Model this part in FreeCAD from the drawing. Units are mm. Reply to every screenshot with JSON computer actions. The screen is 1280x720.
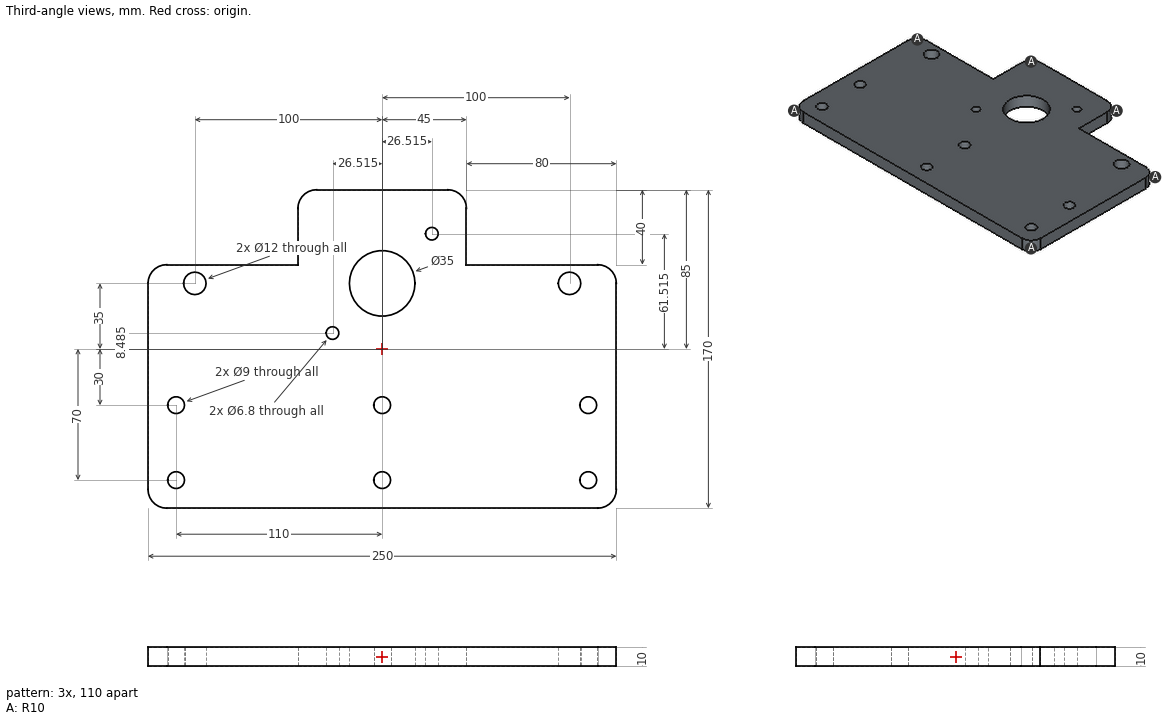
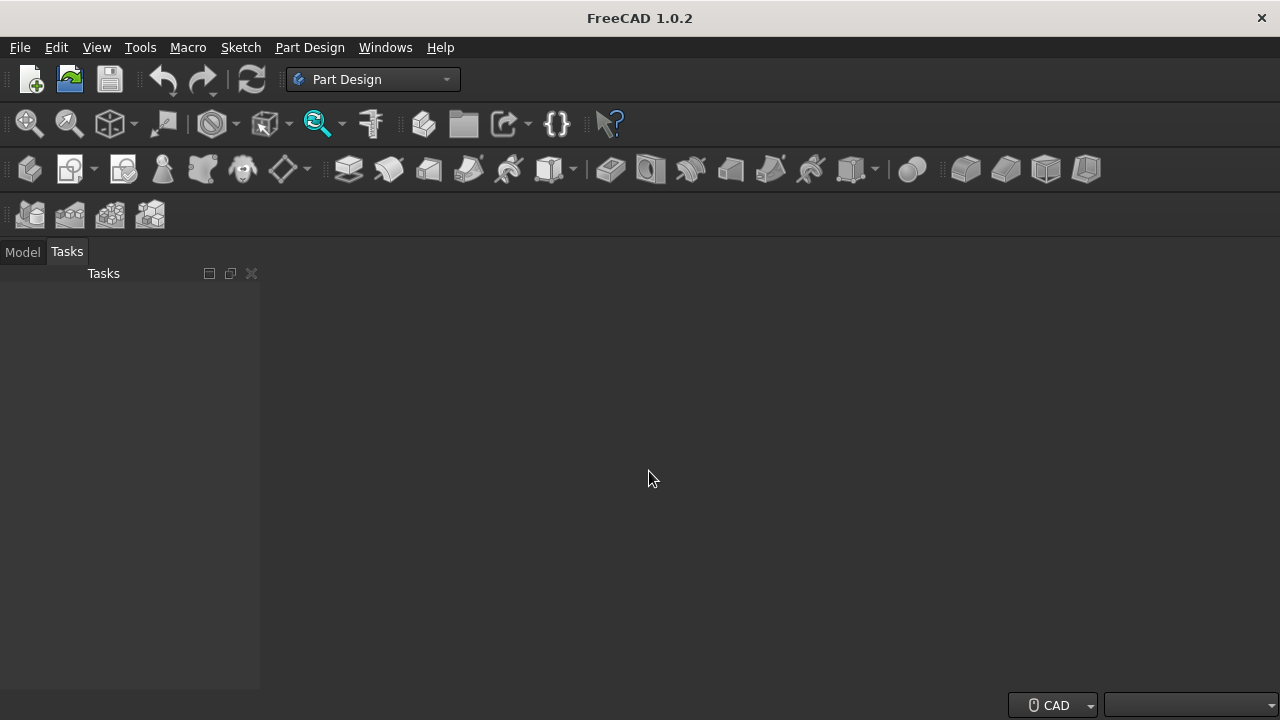
{"action": "left_click", "coordinate": [30, 80]}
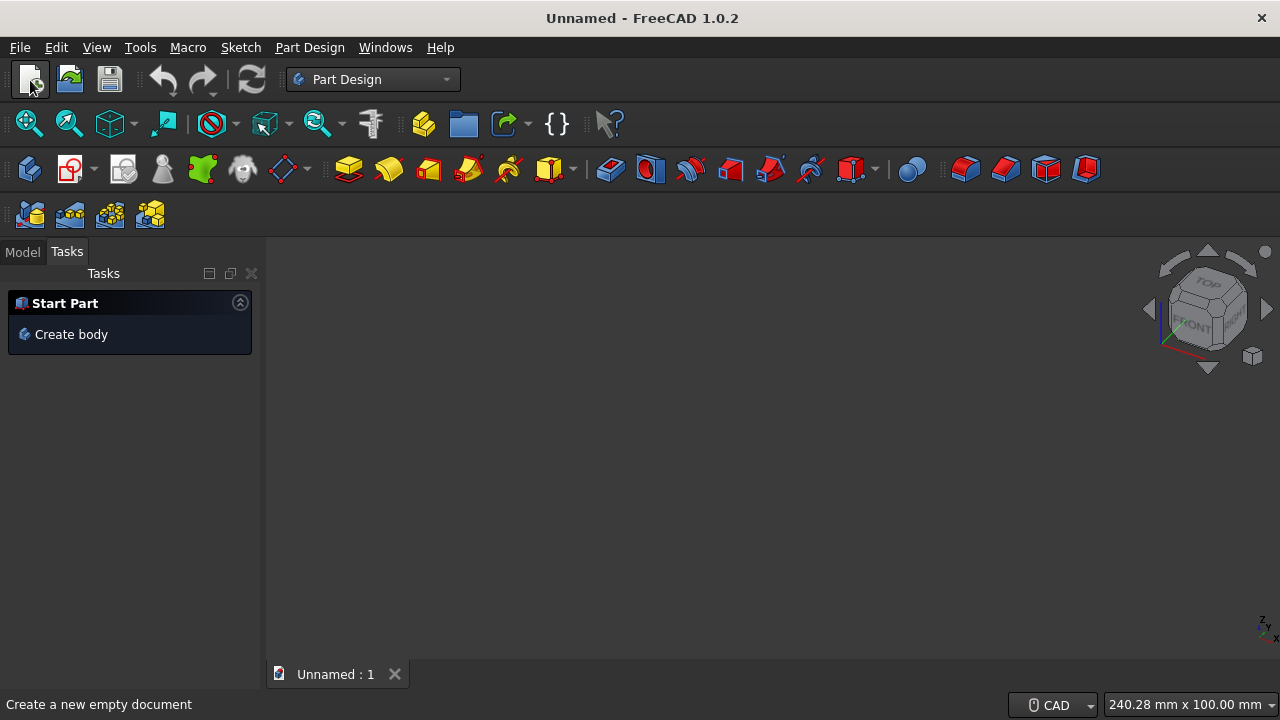
{"action": "left_click", "coordinate": [70, 170]}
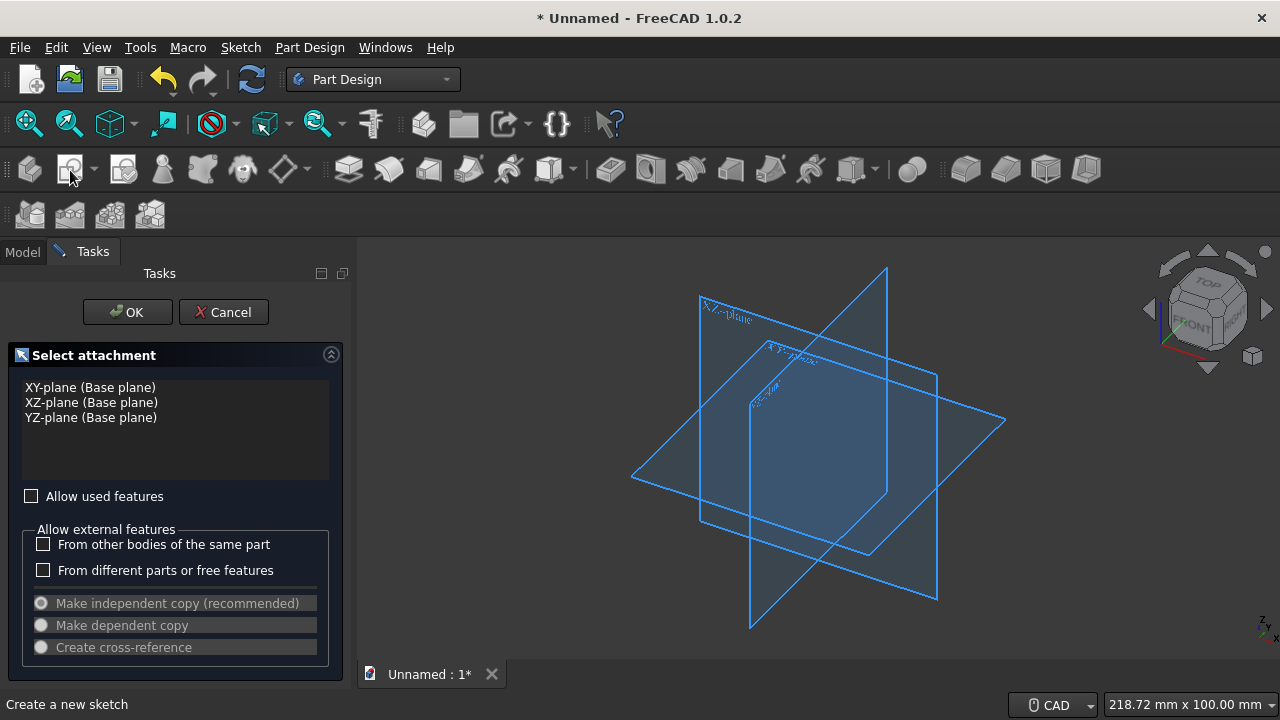
{"action": "left_click", "coordinate": [82, 388]}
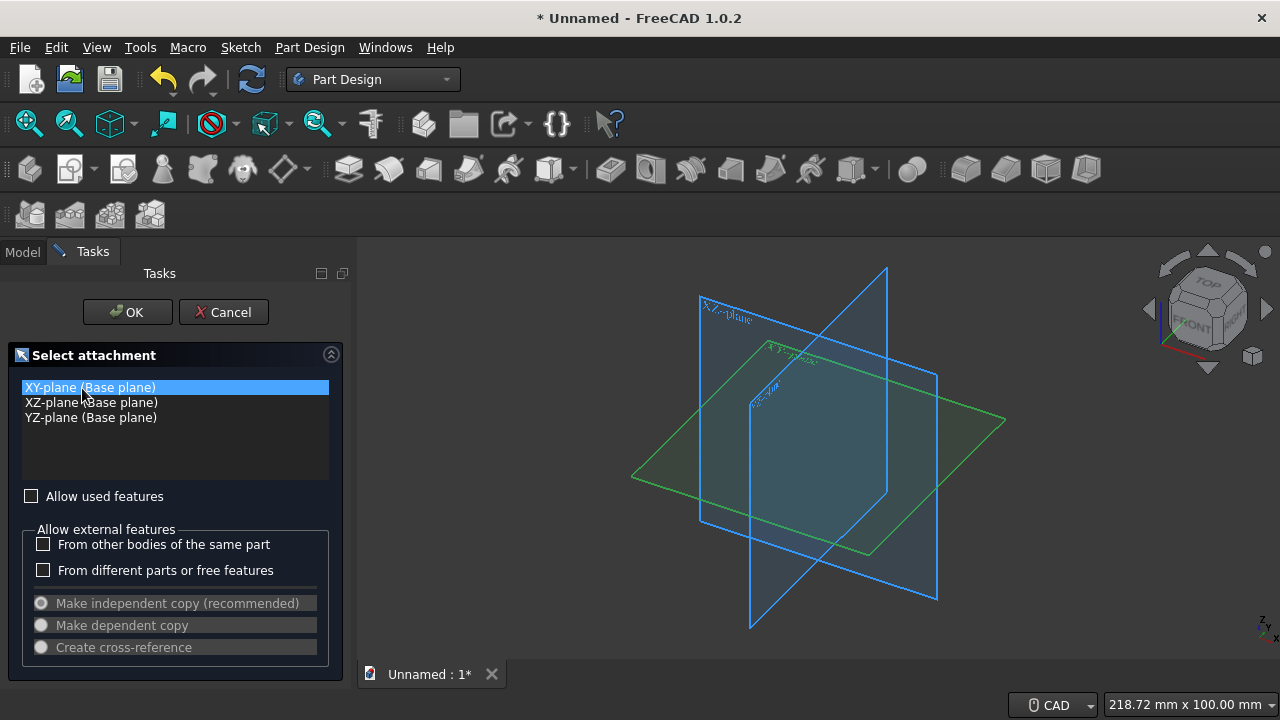
{"action": "left_click", "coordinate": [128, 312]}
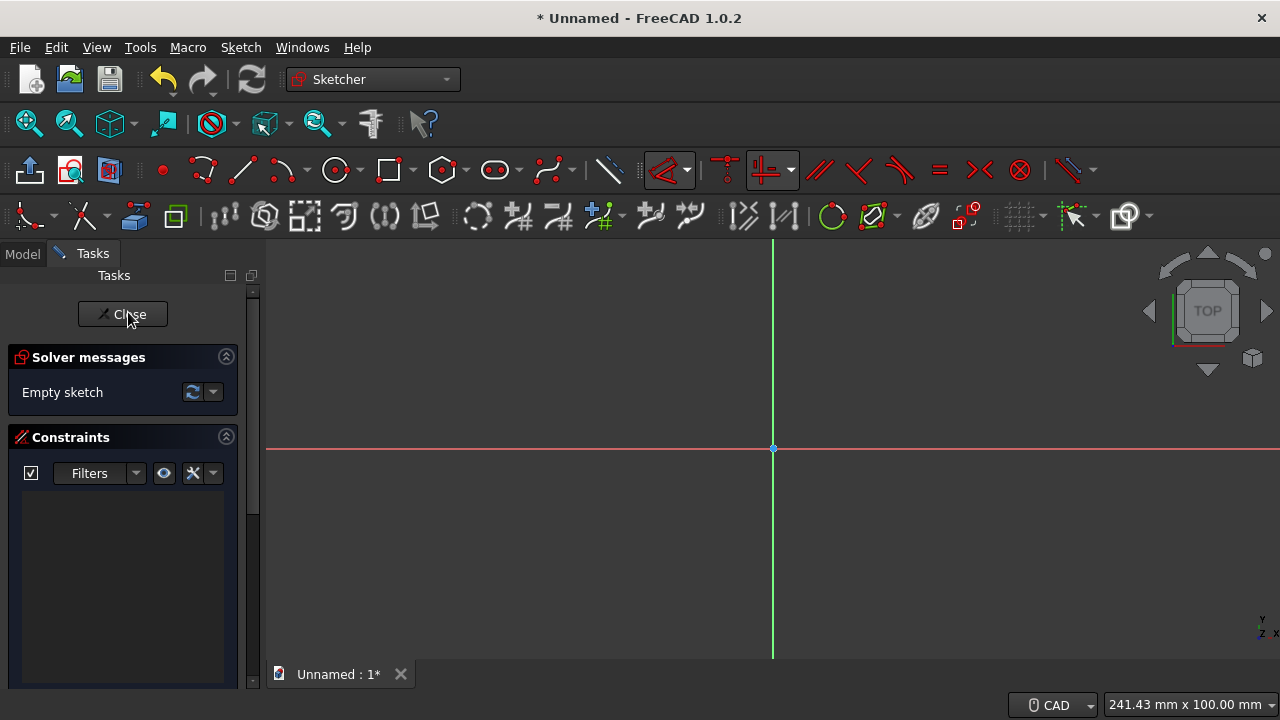
{"action": "scroll", "coordinate": [665, 449], "scroll_direction": "down", "scroll_amount": 5}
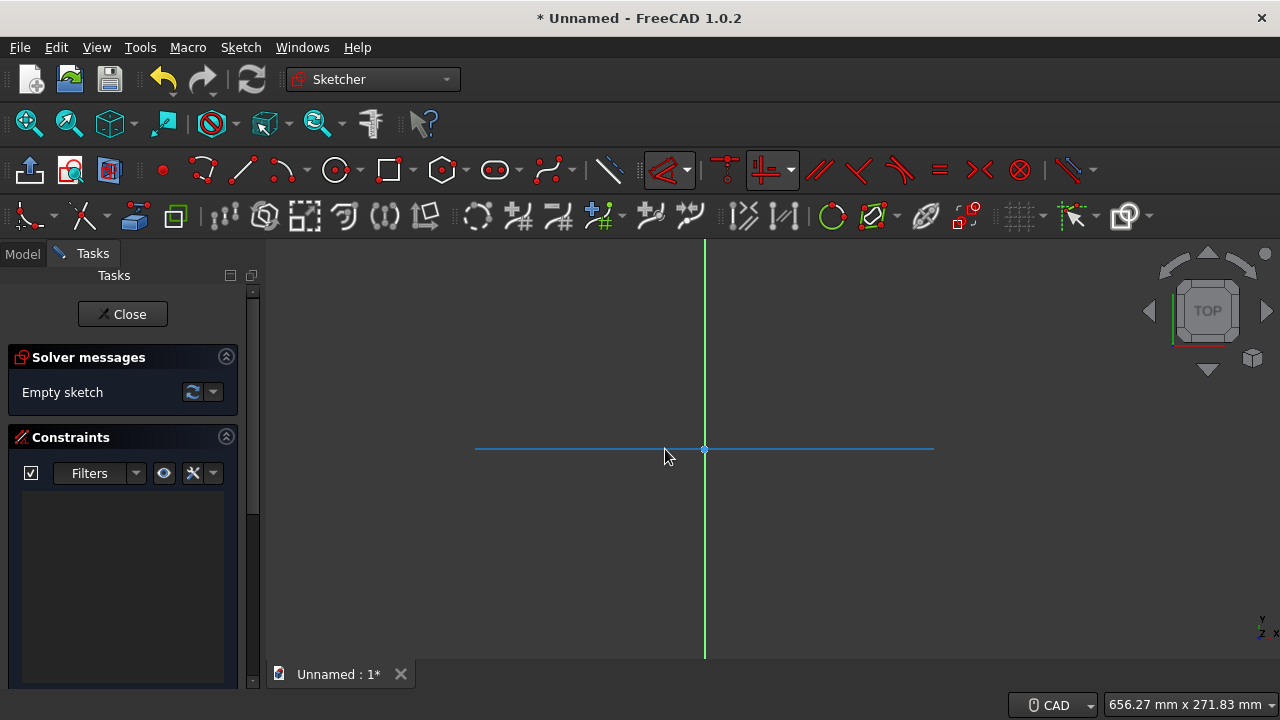
{"action": "key", "text": "g v"}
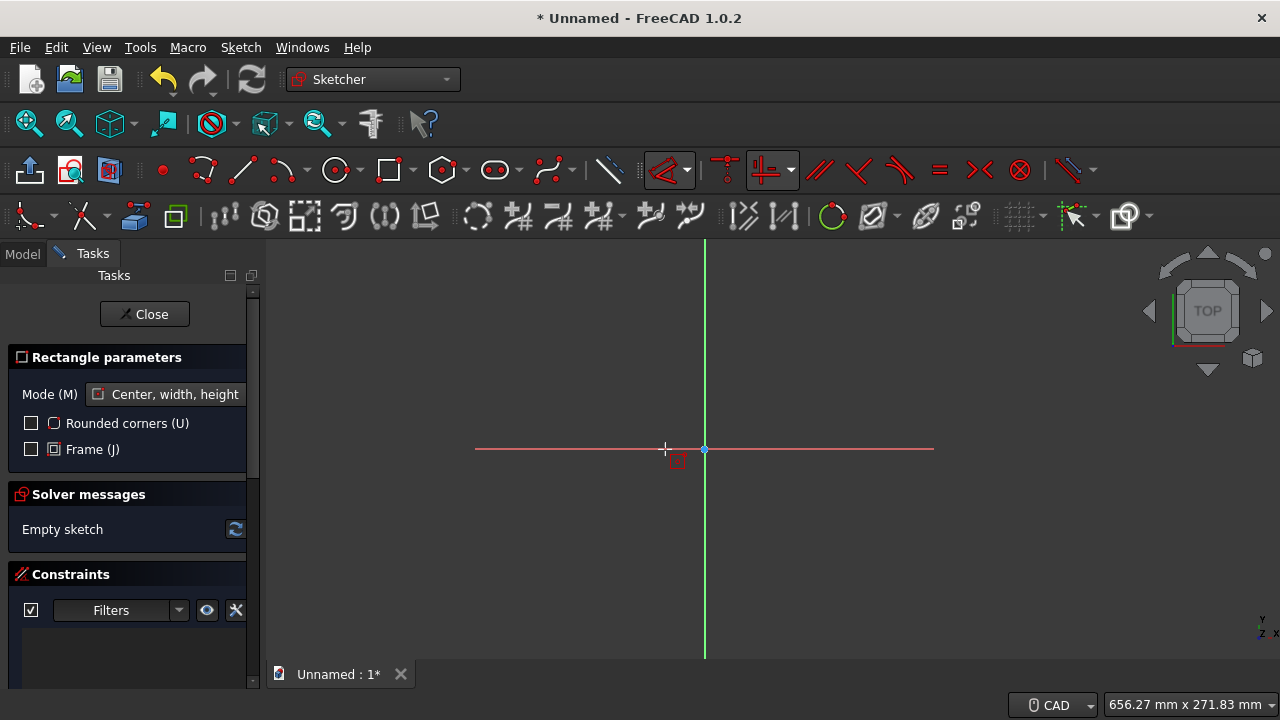
{"action": "left_click", "coordinate": [705, 449]}
{"action": "mouse_move", "coordinate": [898, 318]}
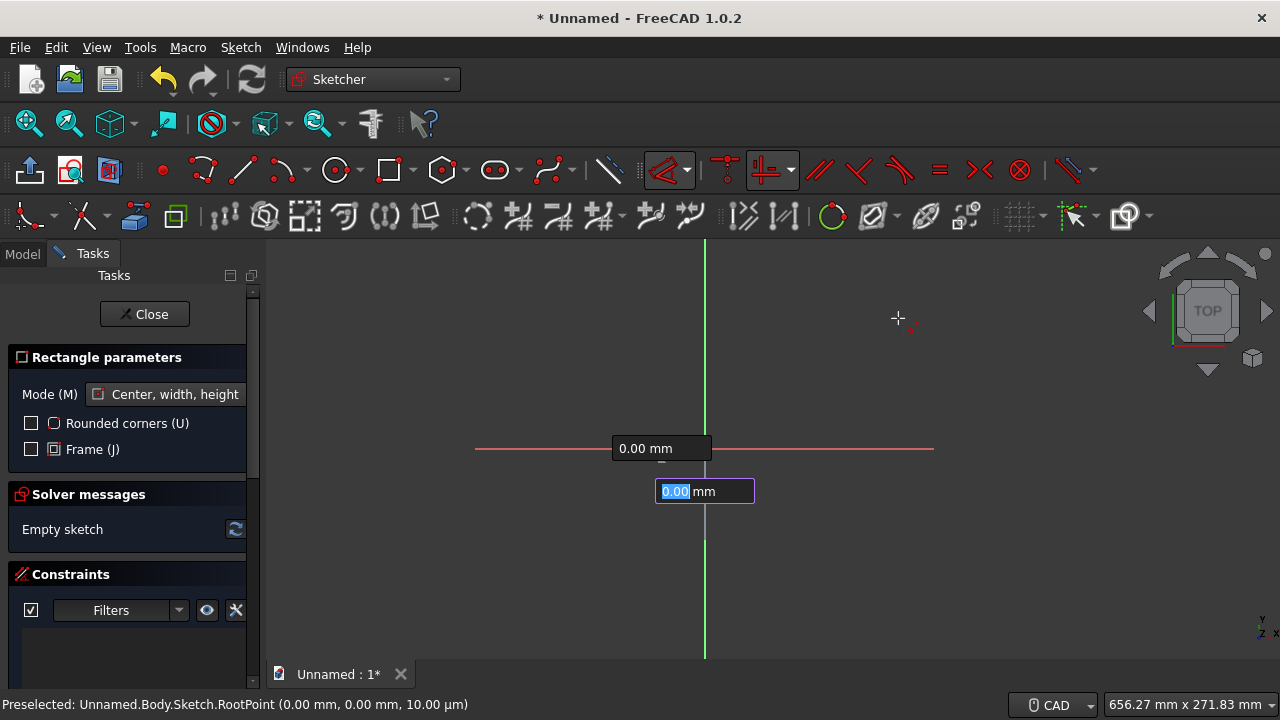
{"action": "type", "text": "250"}
{"action": "key", "text": "Tab"}
{"action": "type", "text": "170"}
{"action": "key", "text": "Return"}
{"action": "key", "text": "Escape"}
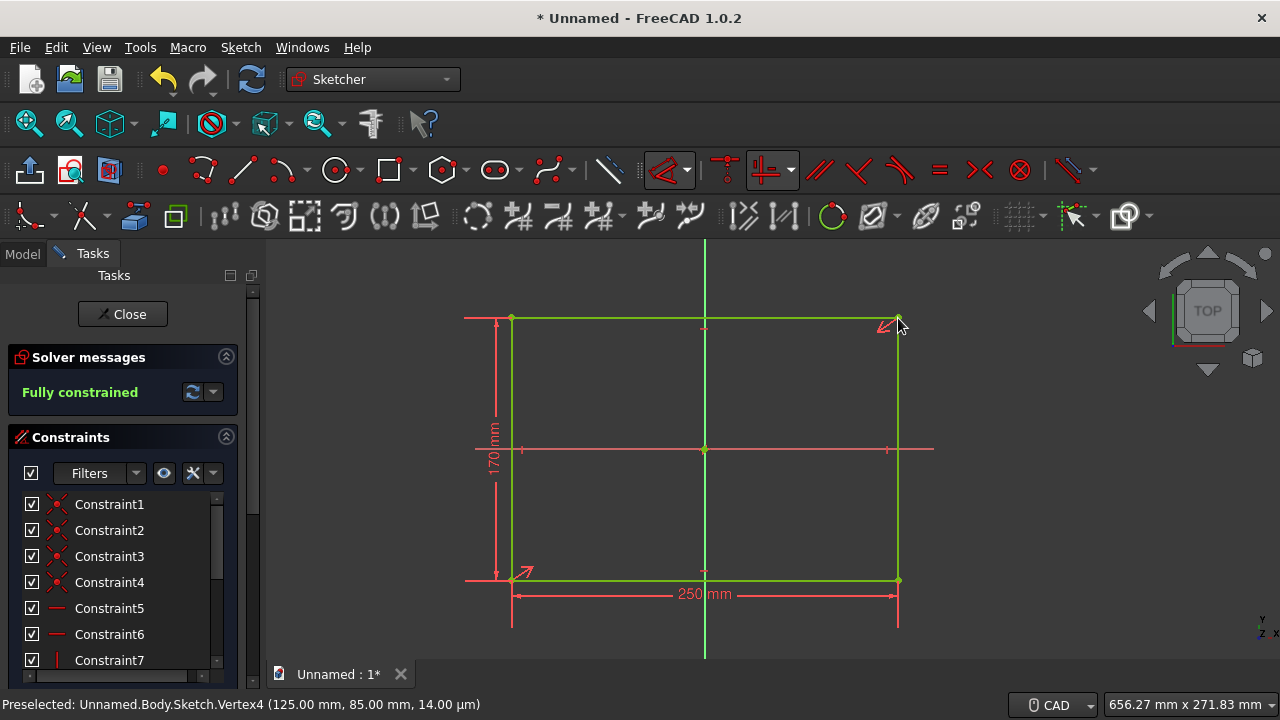
{"action": "left_click", "coordinate": [123, 314]}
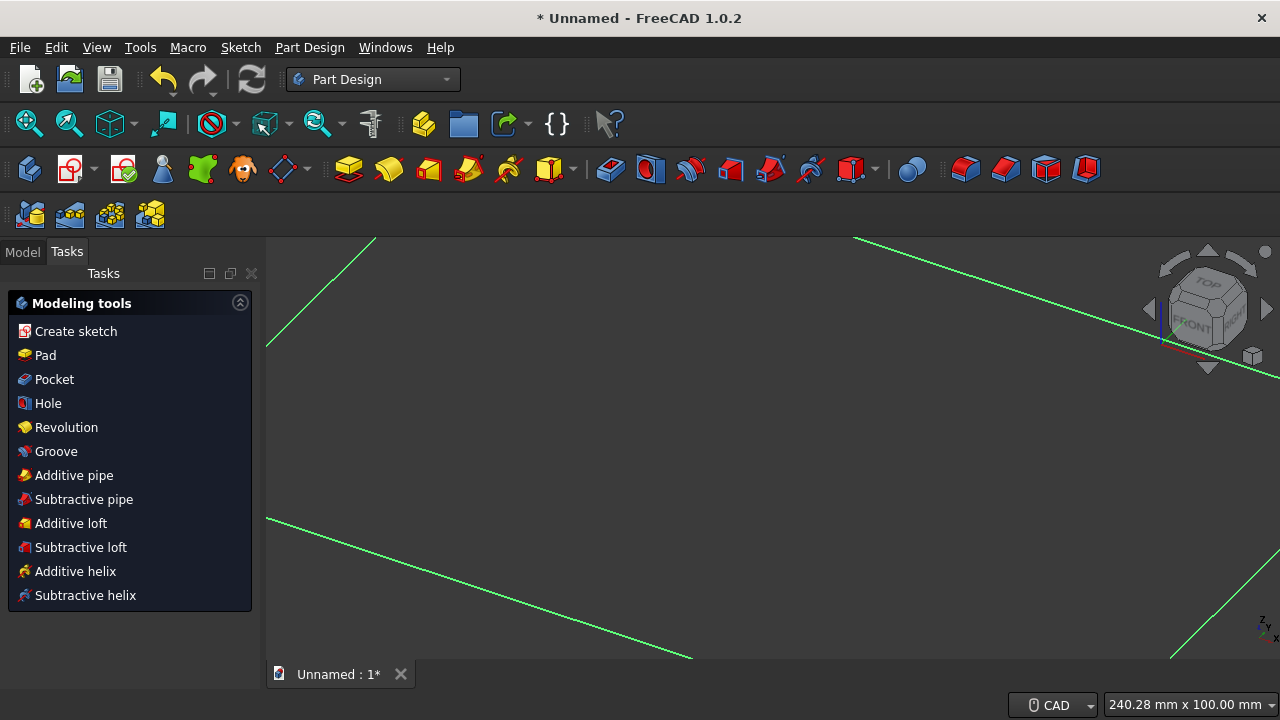
{"action": "left_click", "coordinate": [350, 170]}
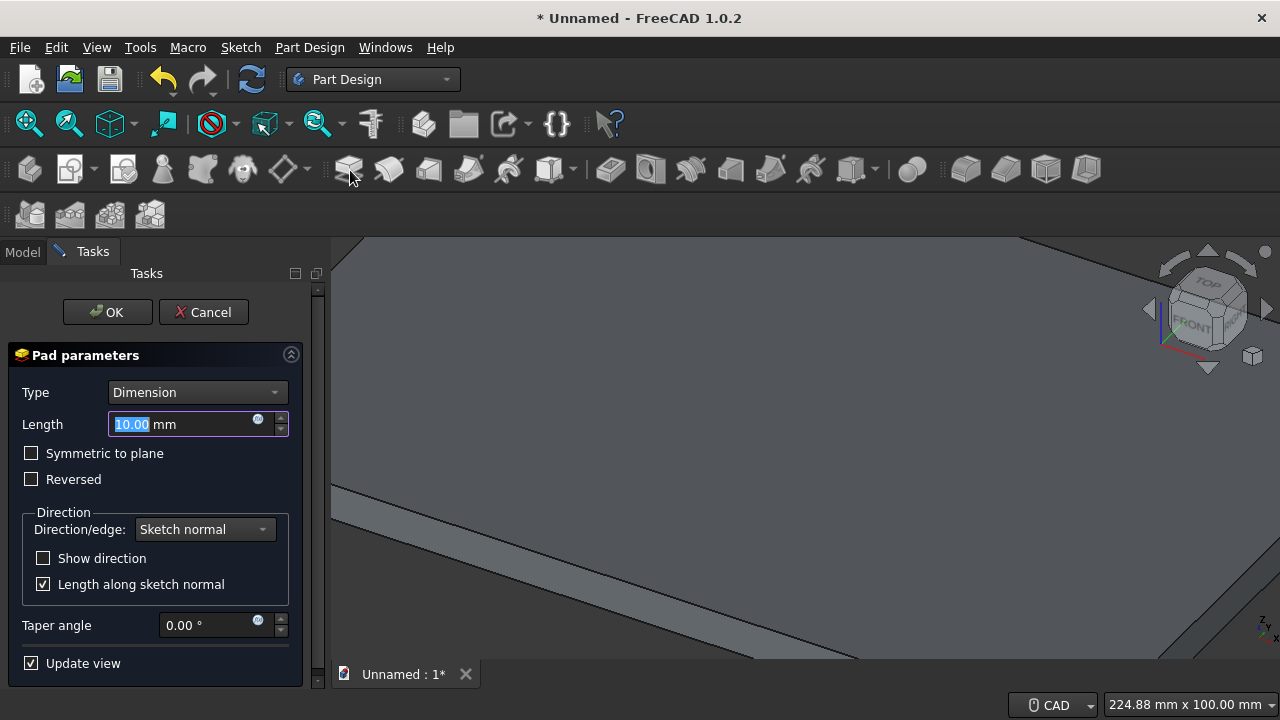
{"action": "type", "text": "10"}
{"action": "key", "text": "Tab"}